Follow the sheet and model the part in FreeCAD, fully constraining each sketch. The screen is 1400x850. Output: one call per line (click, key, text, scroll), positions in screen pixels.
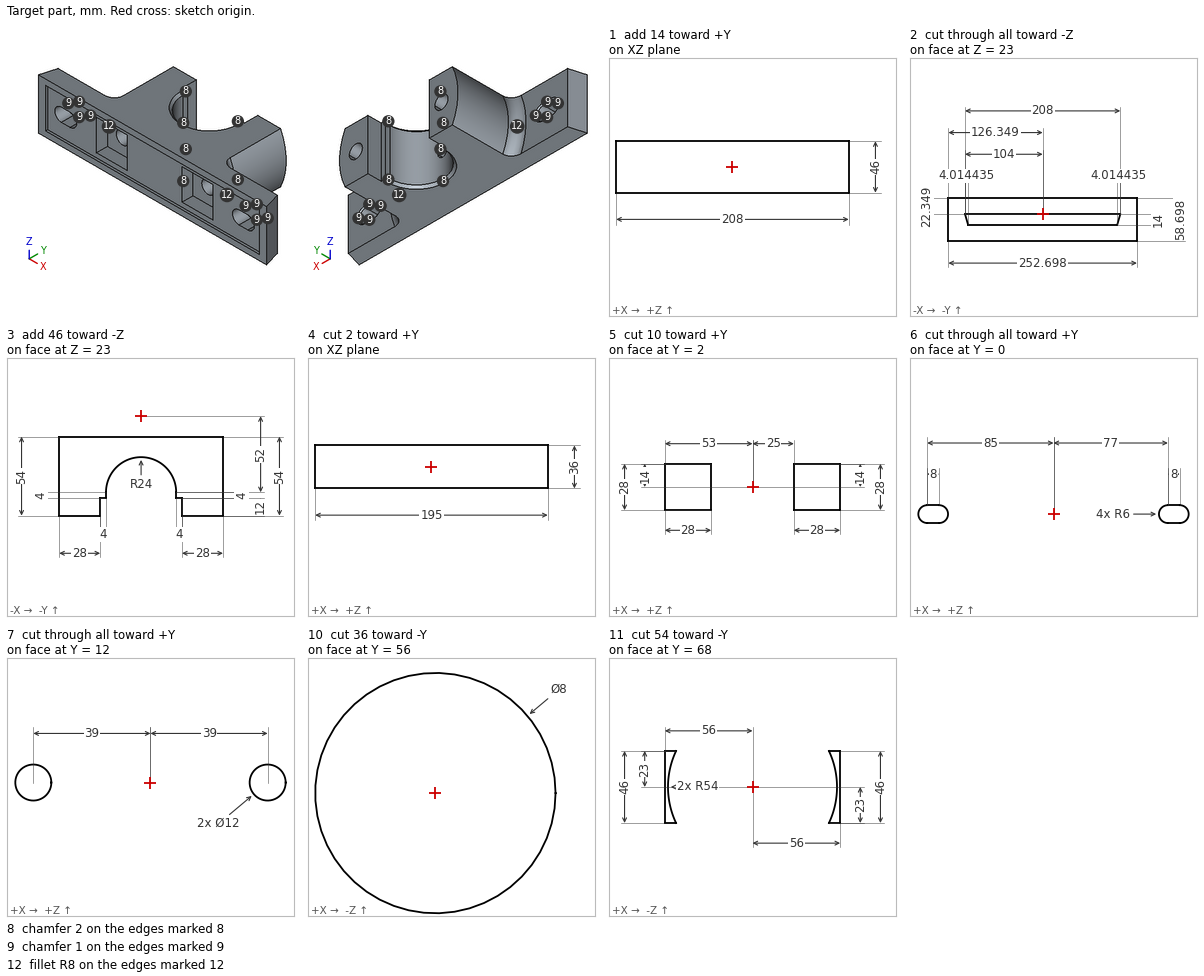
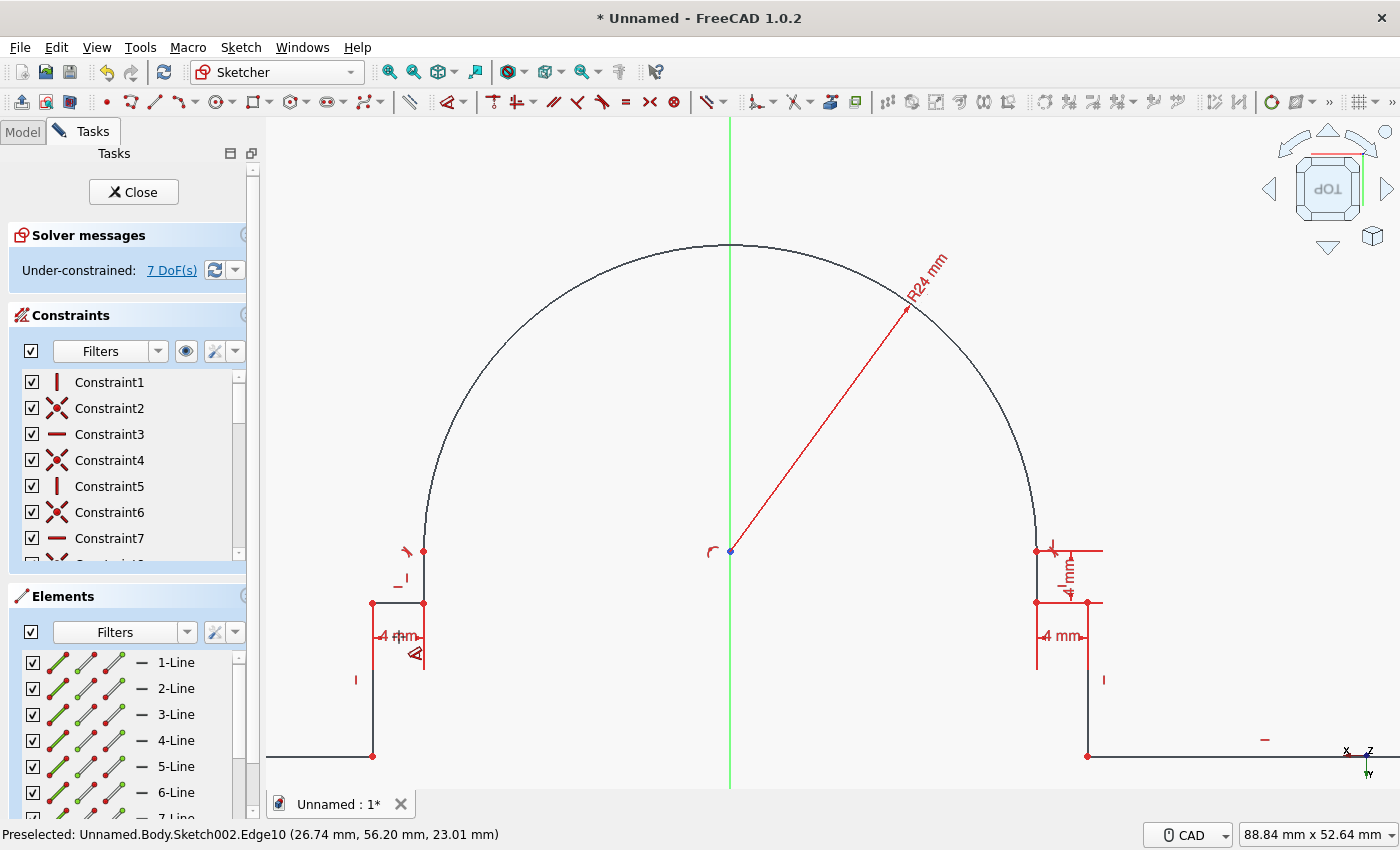
click(424, 588)
click(390, 577)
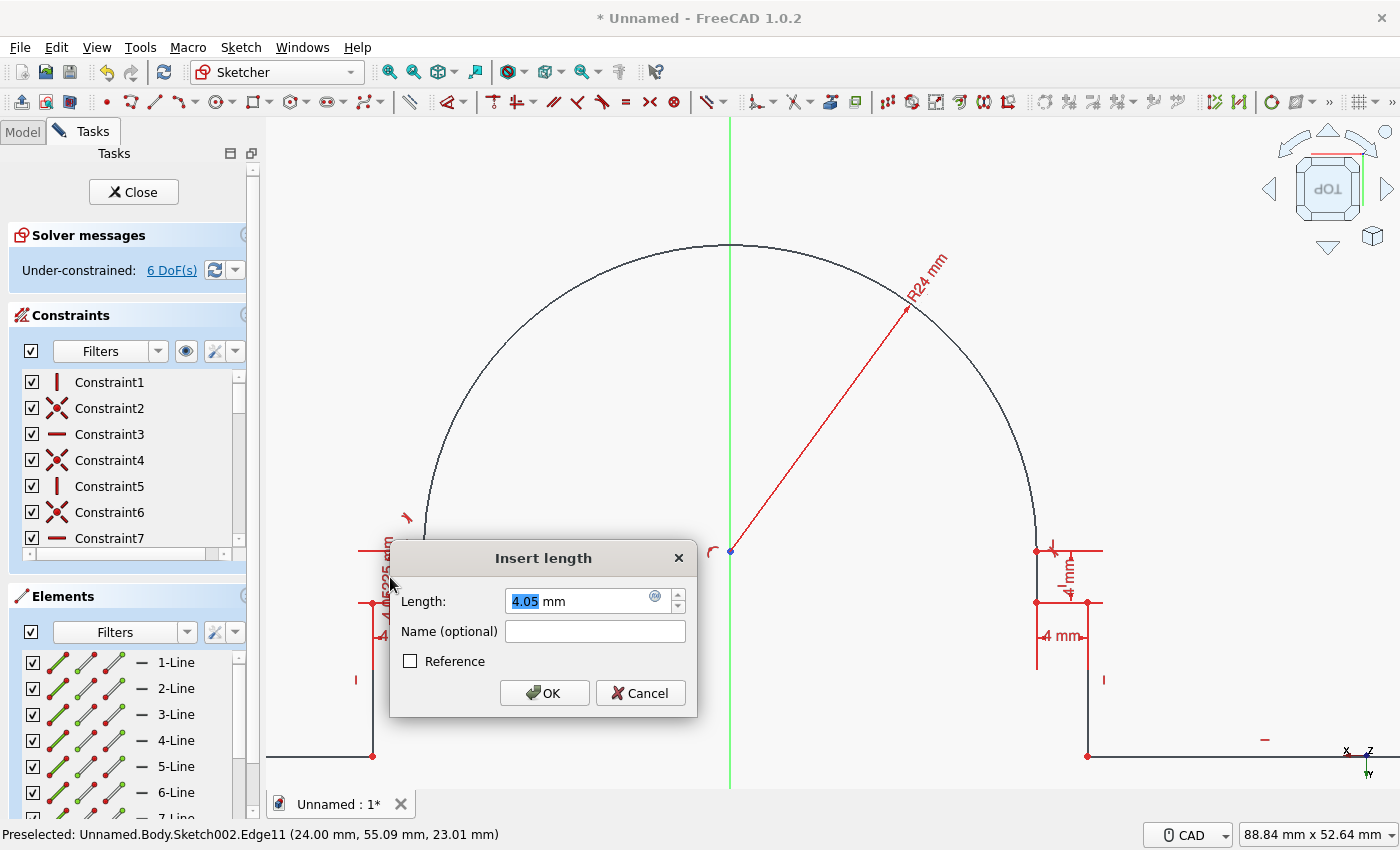
text(4)
key(Return)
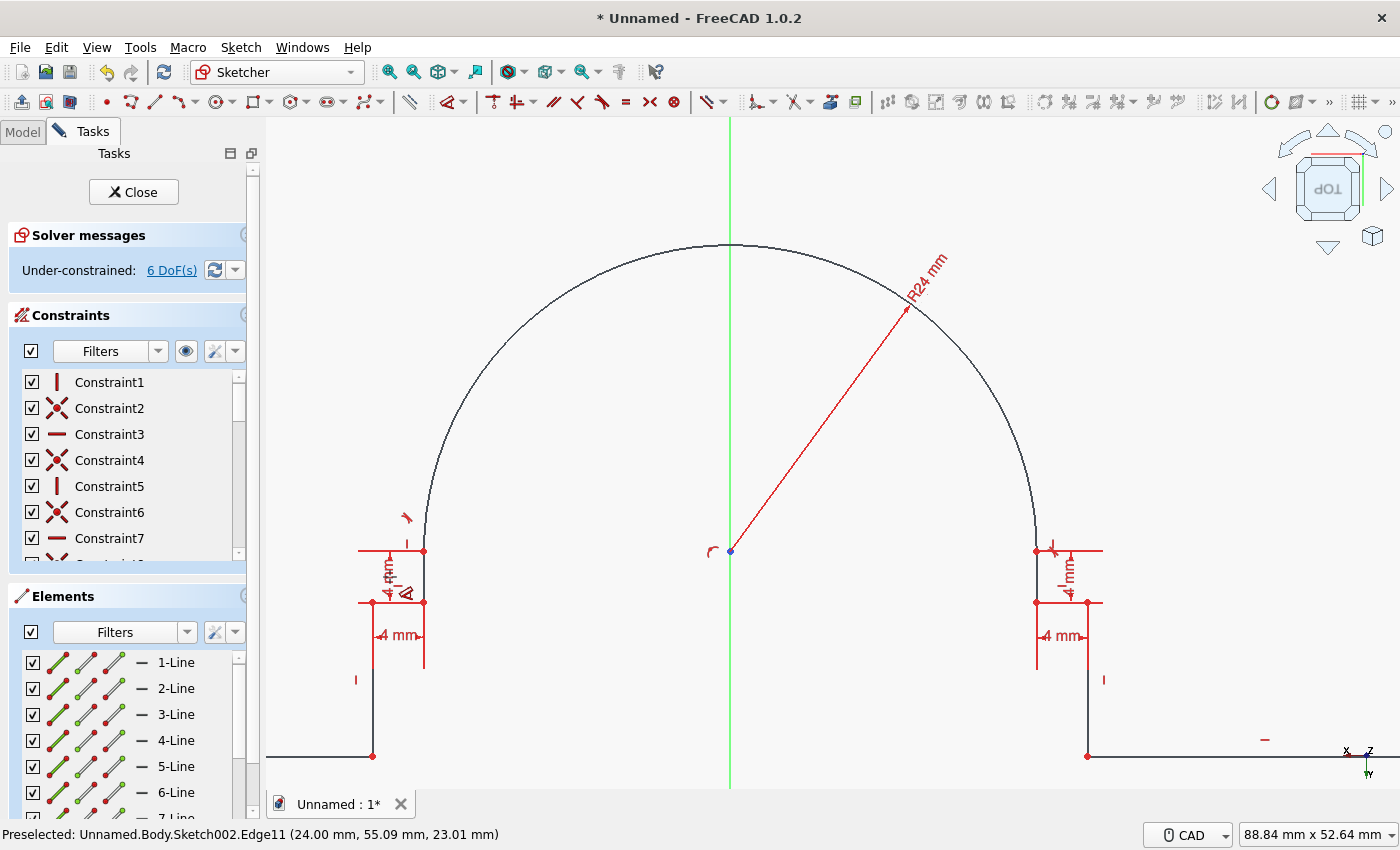
click(1088, 649)
click(1122, 680)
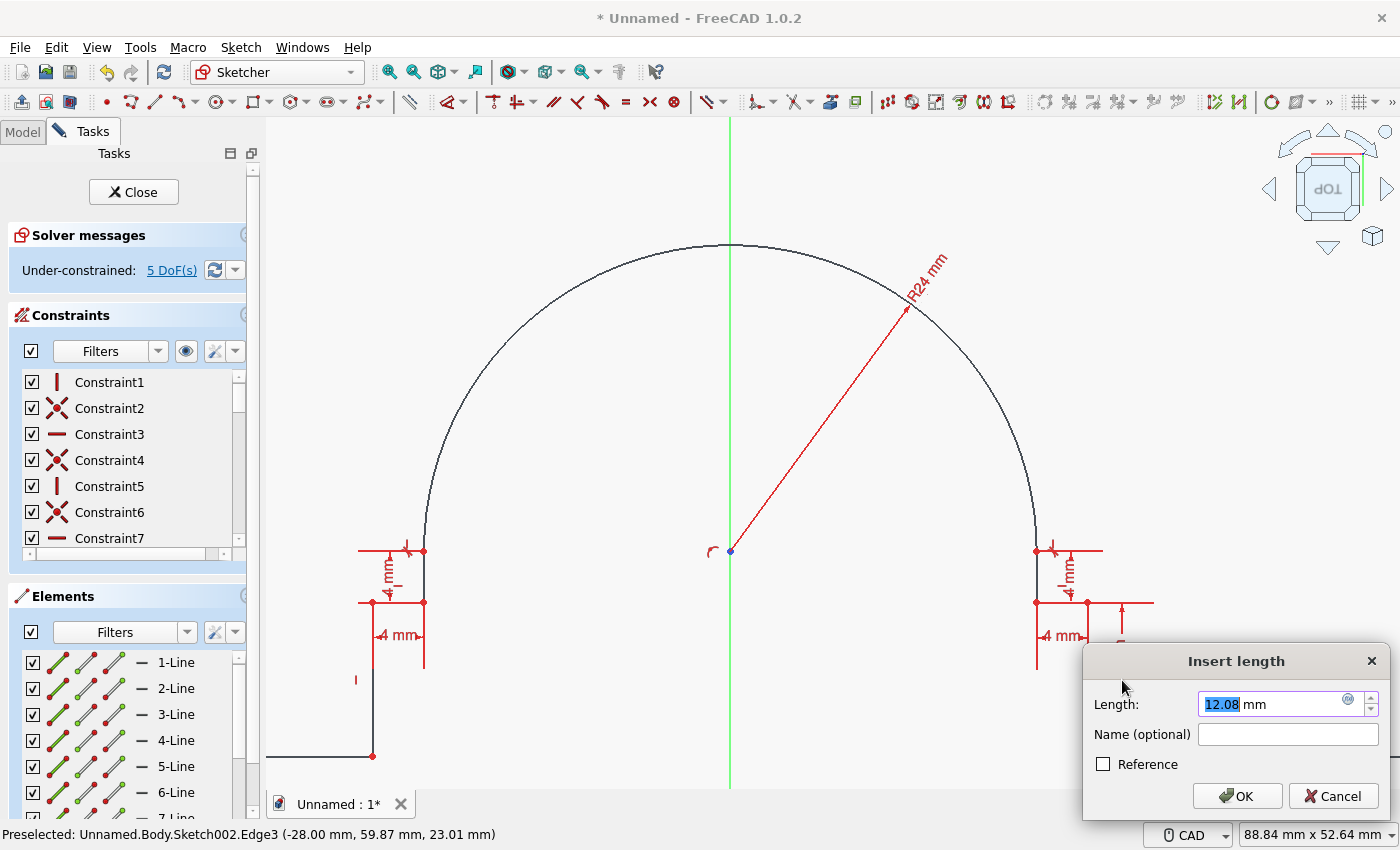
text(12)
key(Return)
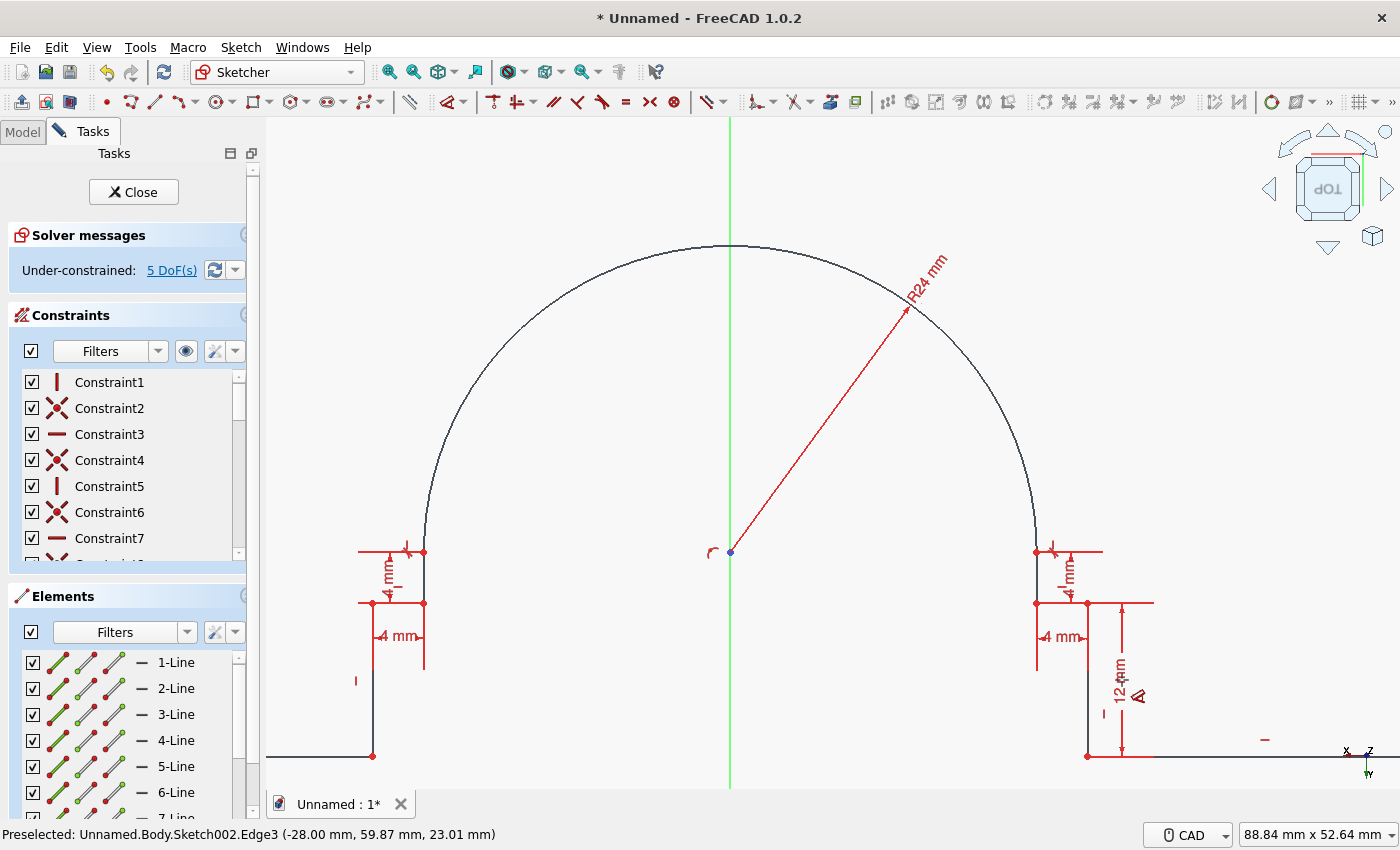
click(1195, 757)
click(1161, 723)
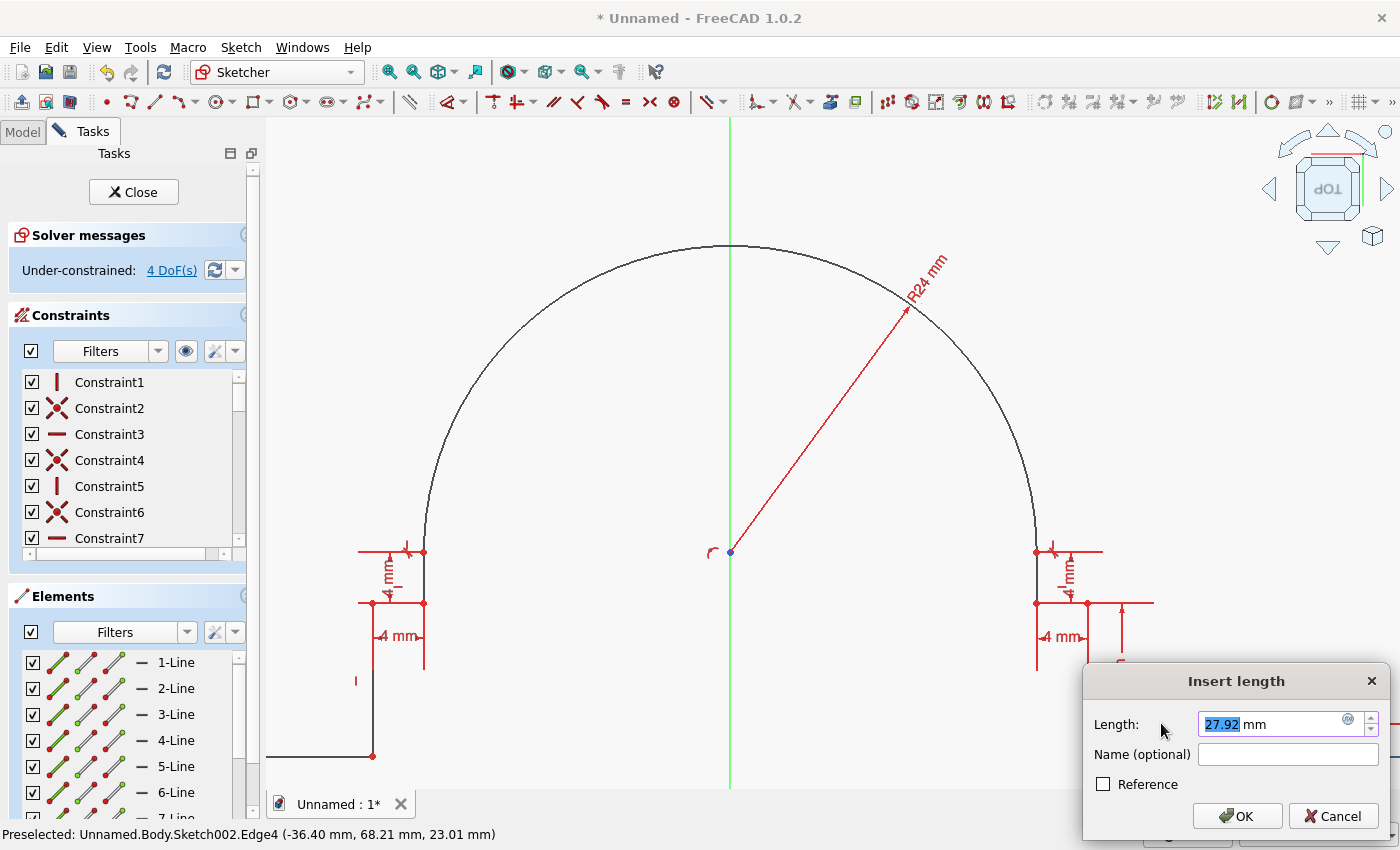
text(28)
key(Return)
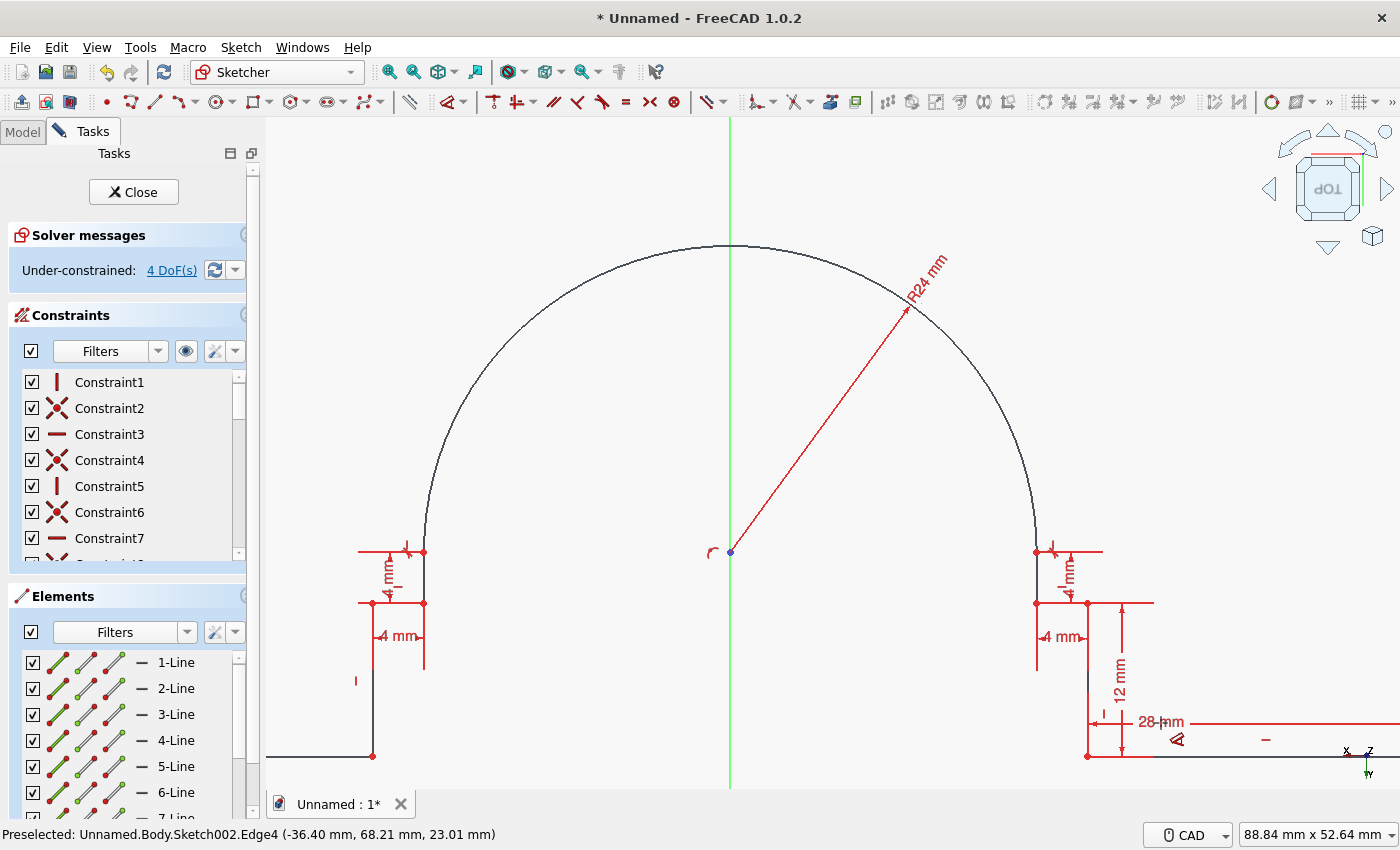
scroll(792, 562, down, 4)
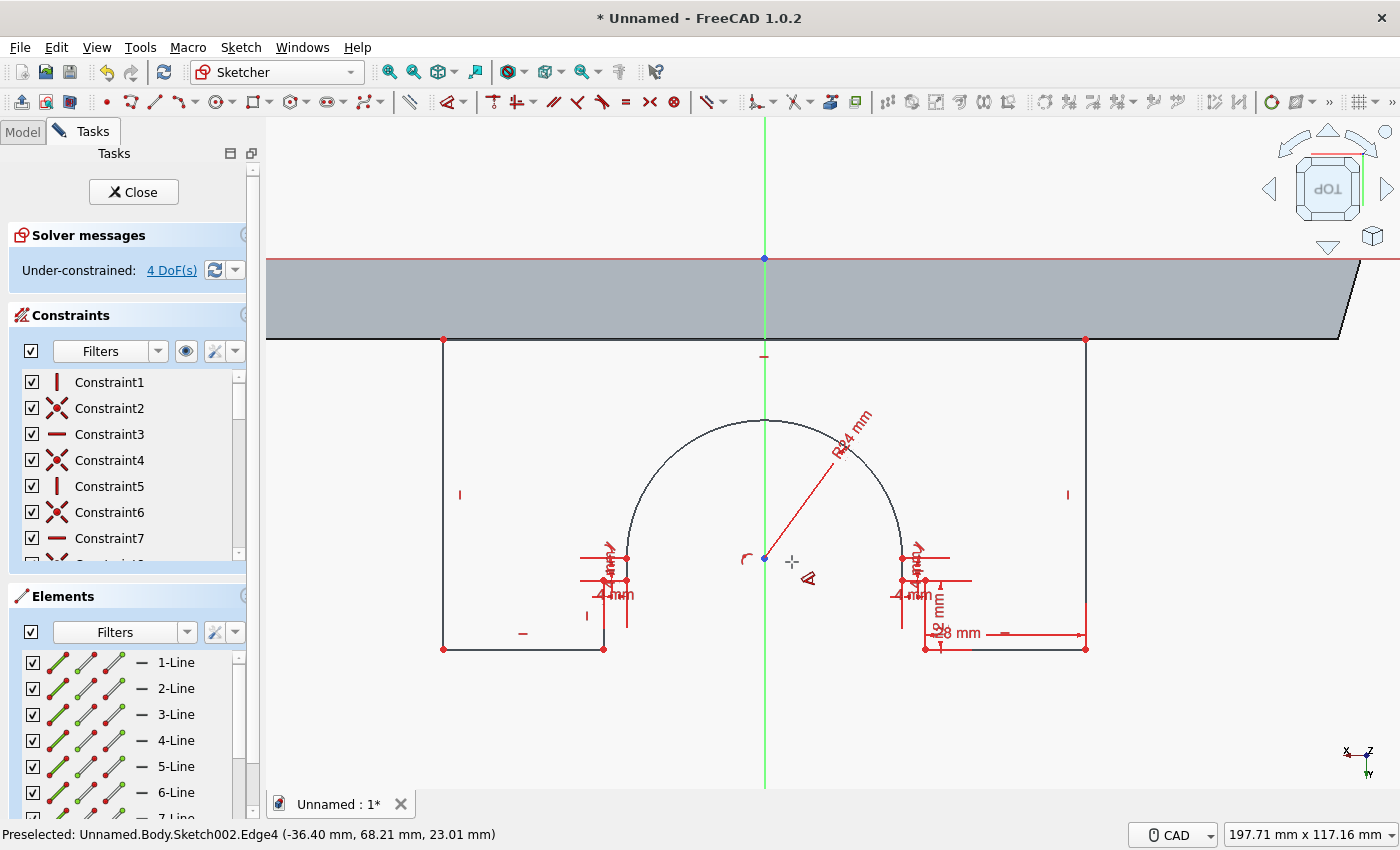
click(1086, 557)
click(1120, 495)